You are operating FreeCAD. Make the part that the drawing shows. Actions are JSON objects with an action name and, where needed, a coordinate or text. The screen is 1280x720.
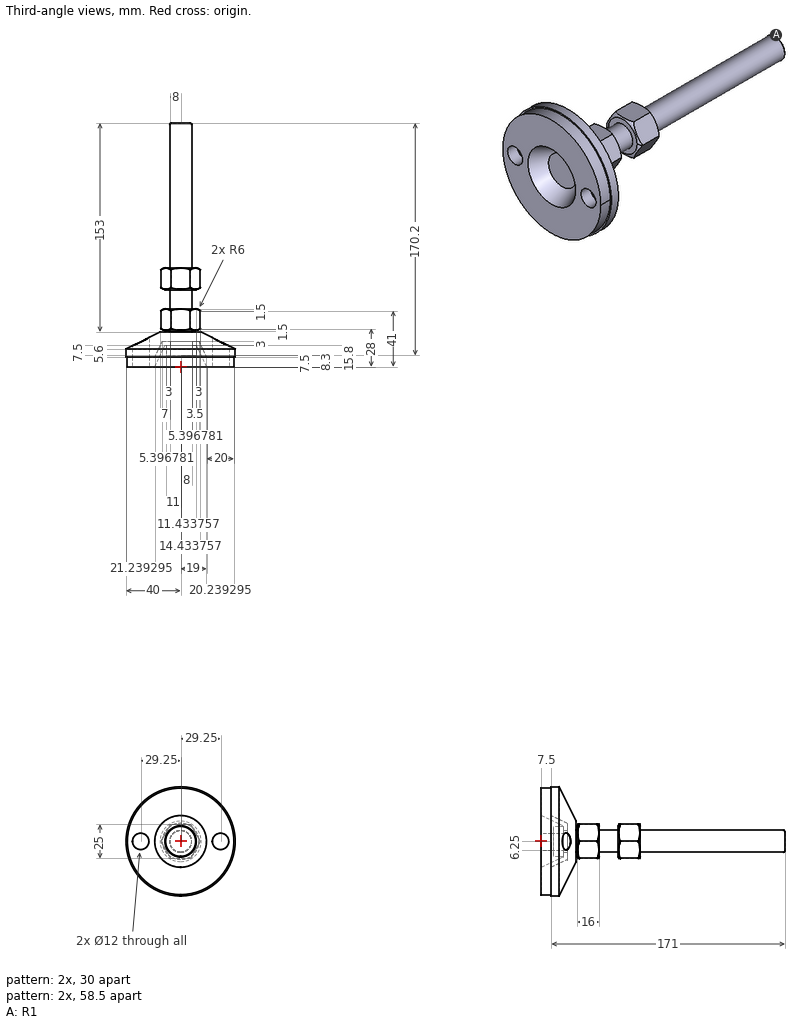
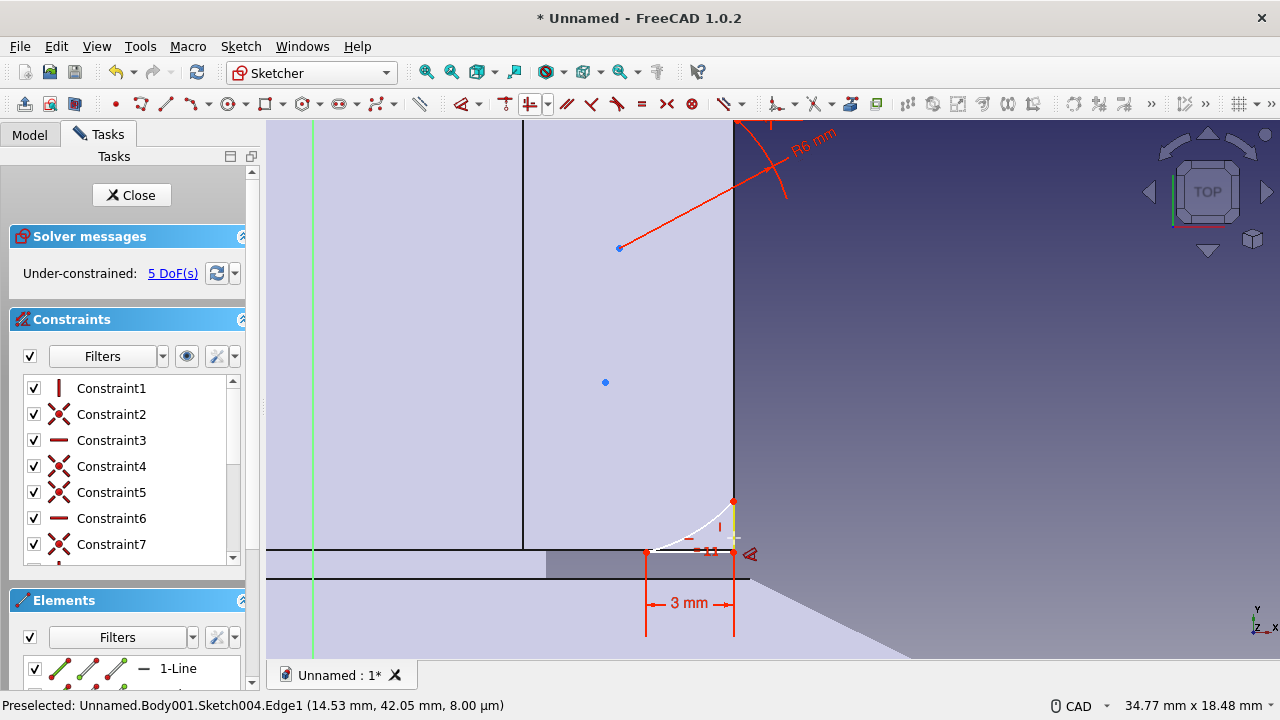
{"action": "left_click", "coordinate": [734, 537]}
{"action": "left_click", "coordinate": [768, 527]}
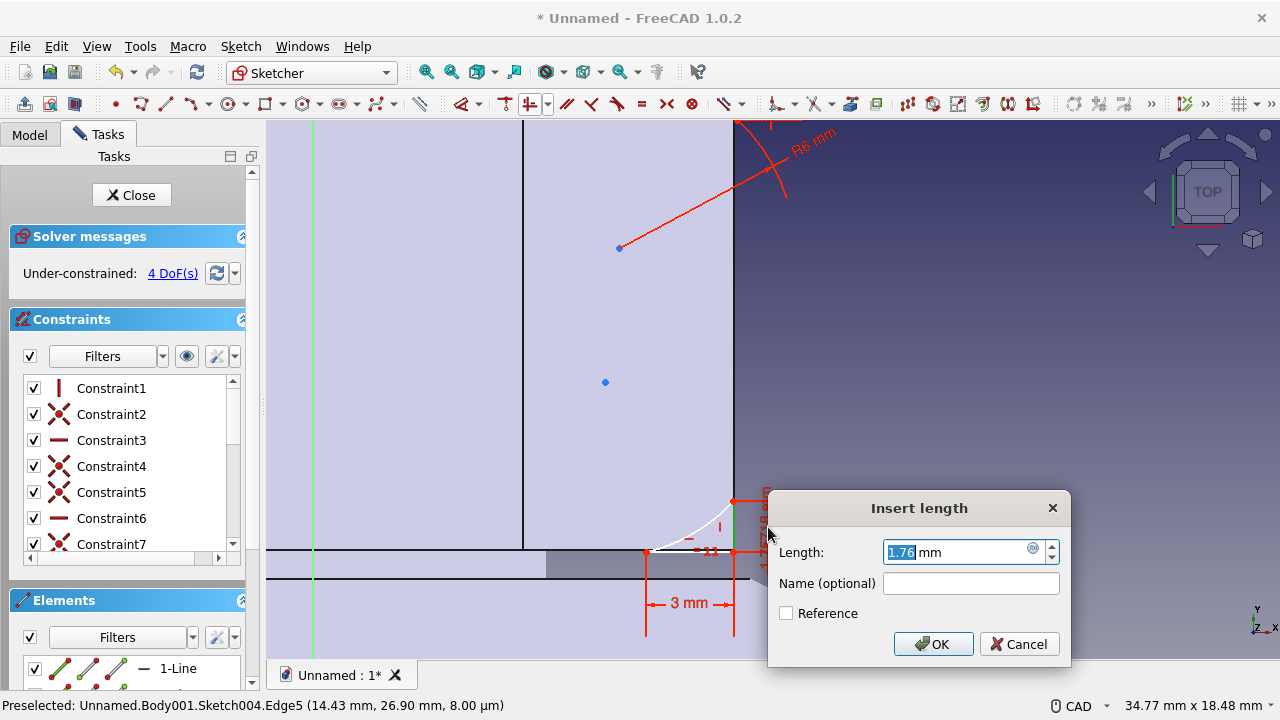
{"action": "type", "text": "1.5"}
{"action": "key", "text": "Return"}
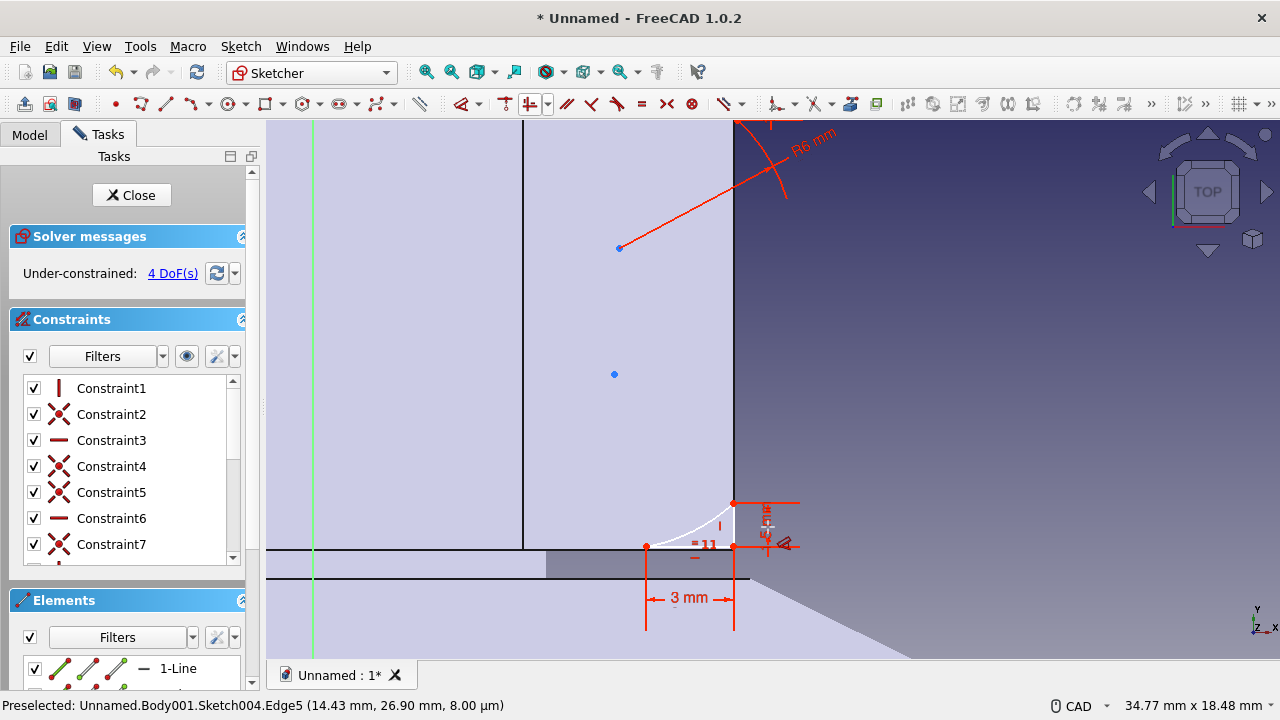
{"action": "scroll", "coordinate": [734, 538], "scroll_direction": "down", "scroll_amount": 2}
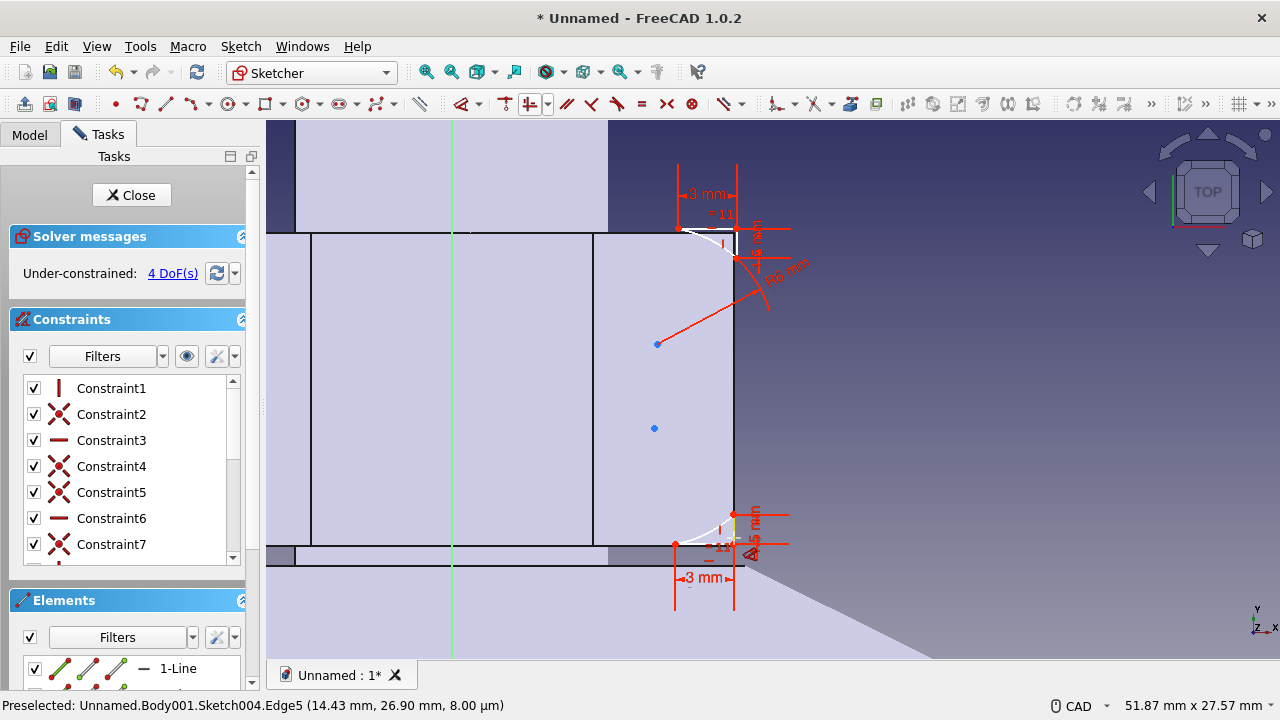
{"action": "left_click", "coordinate": [737, 258]}
{"action": "left_click", "coordinate": [418, 445]}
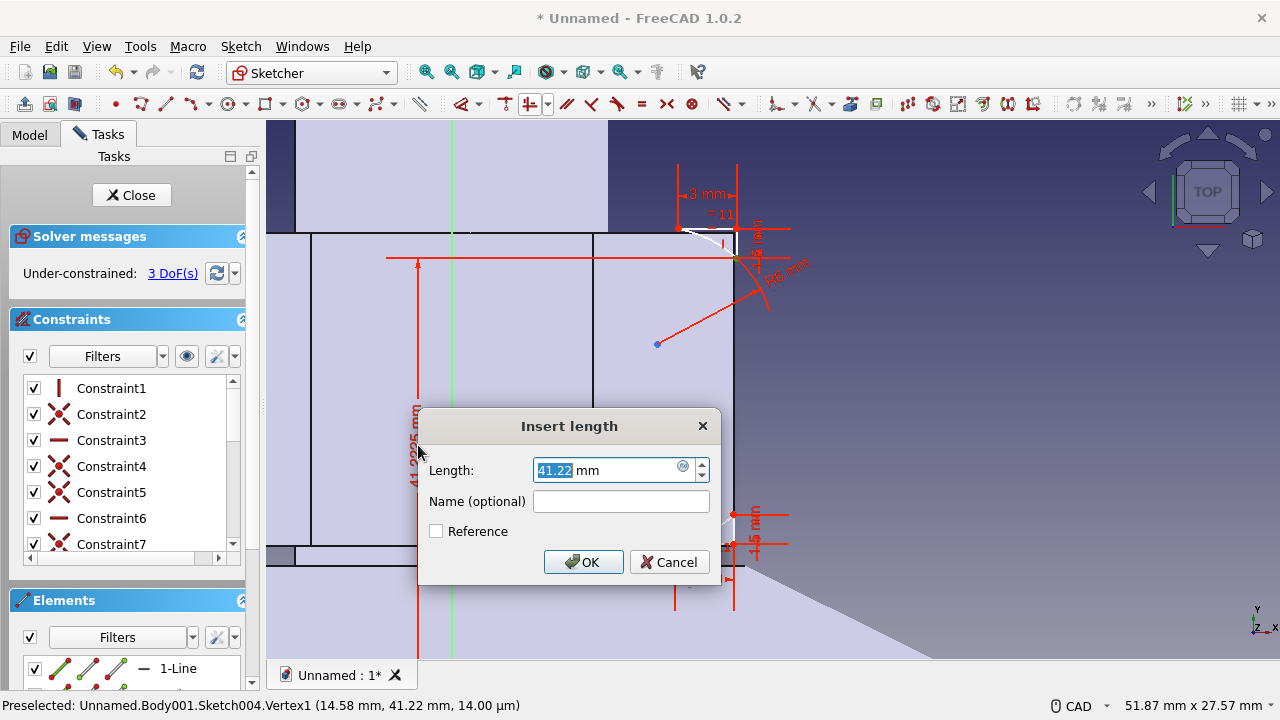
{"action": "type", "text": "41"}
{"action": "key", "text": "Return"}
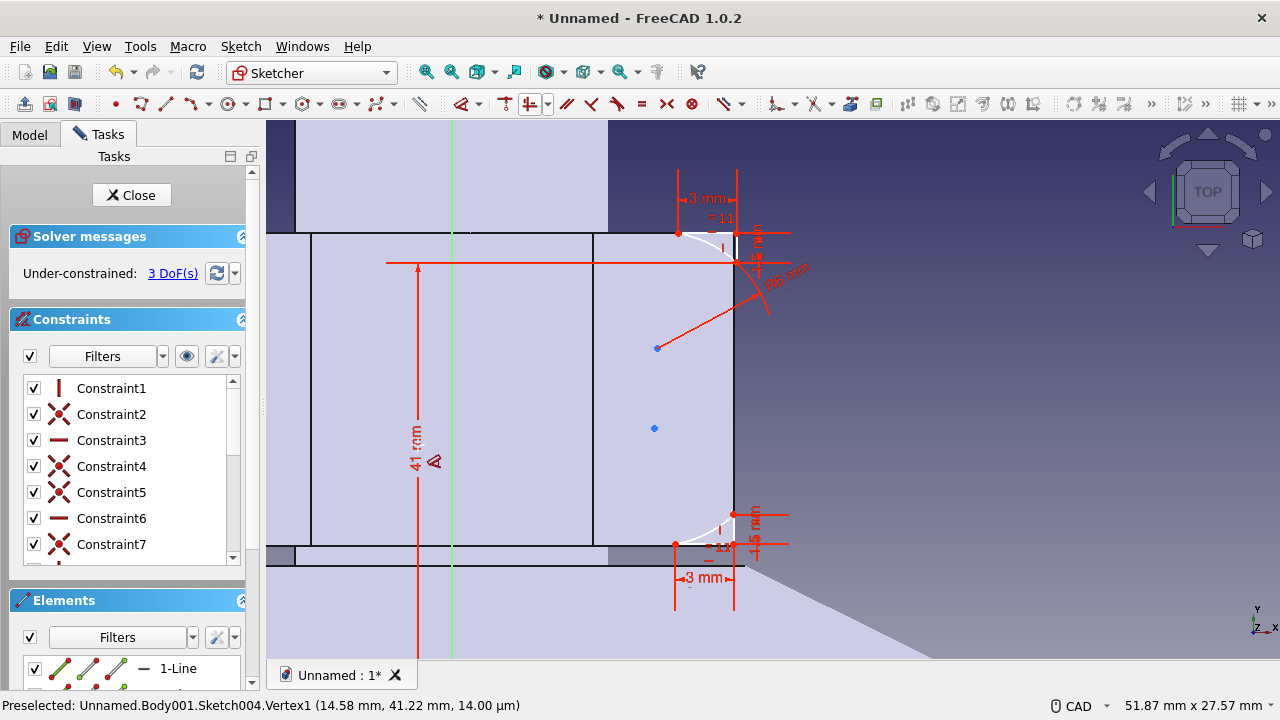
{"action": "left_click", "coordinate": [734, 515]}
{"action": "left_click", "coordinate": [418, 573]}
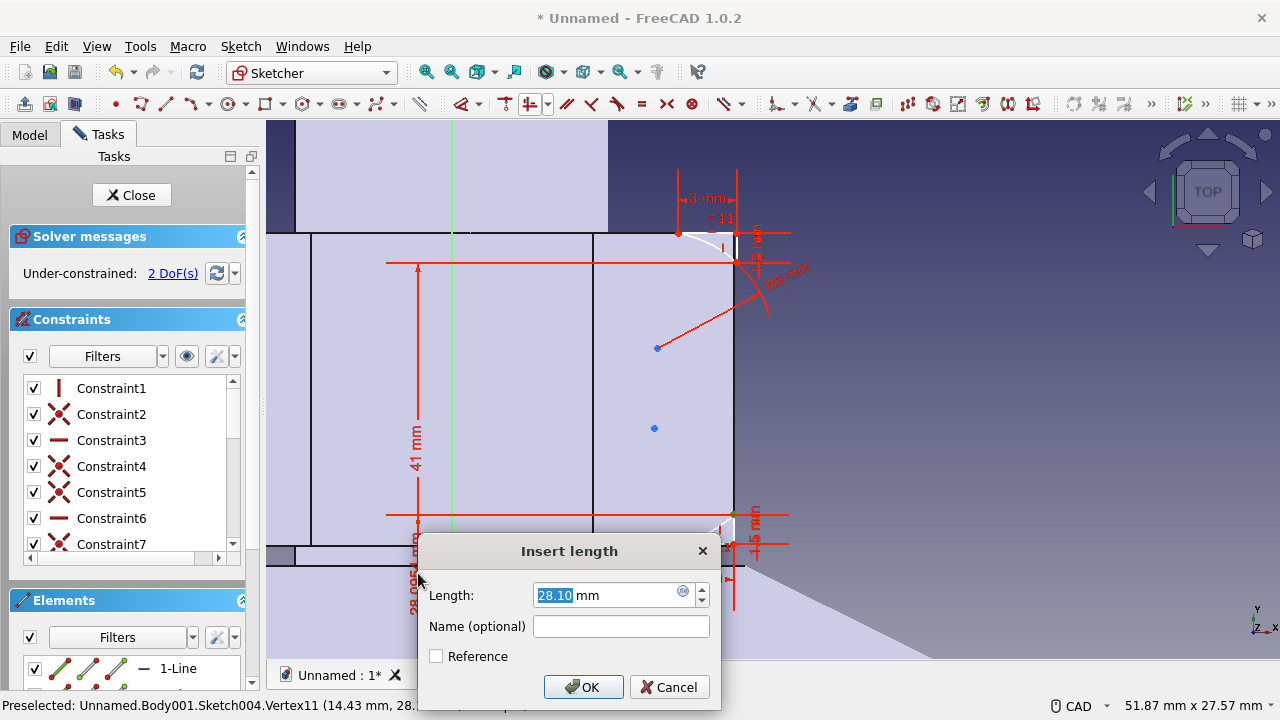
{"action": "type", "text": "28"}
{"action": "key", "text": "Return"}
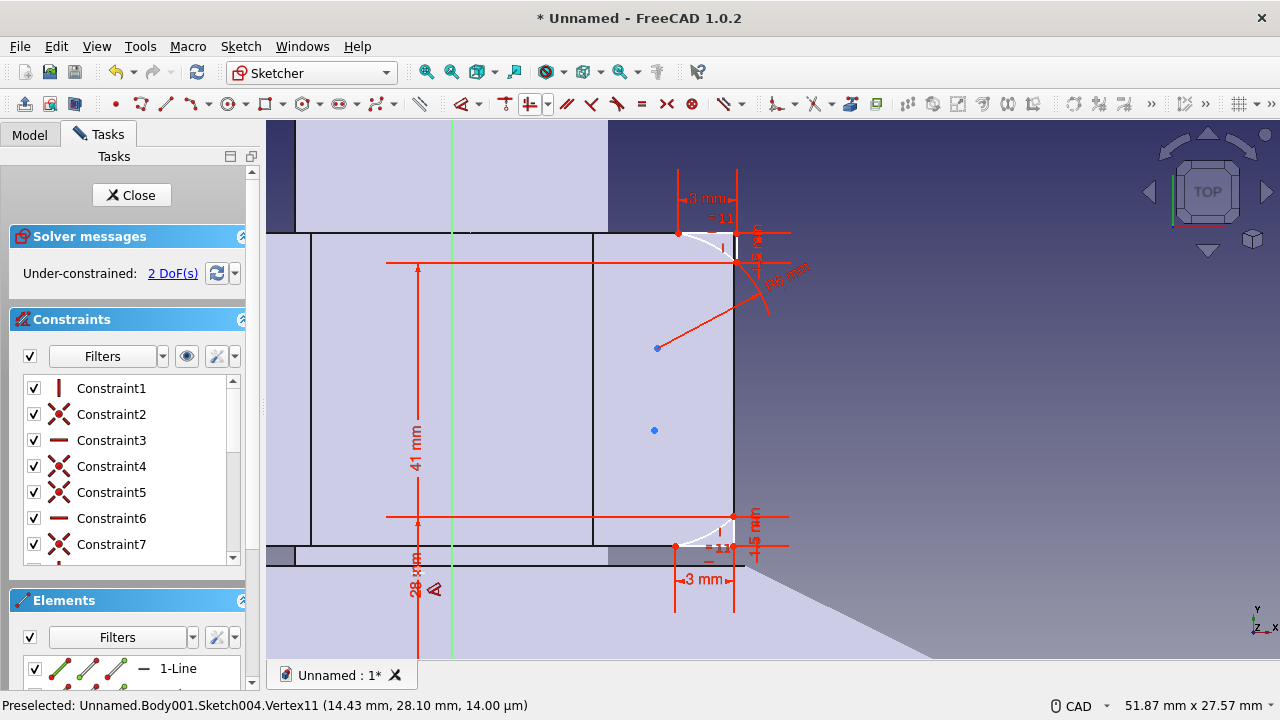
{"action": "left_click", "coordinate": [737, 263]}
{"action": "left_click", "coordinate": [594, 229]}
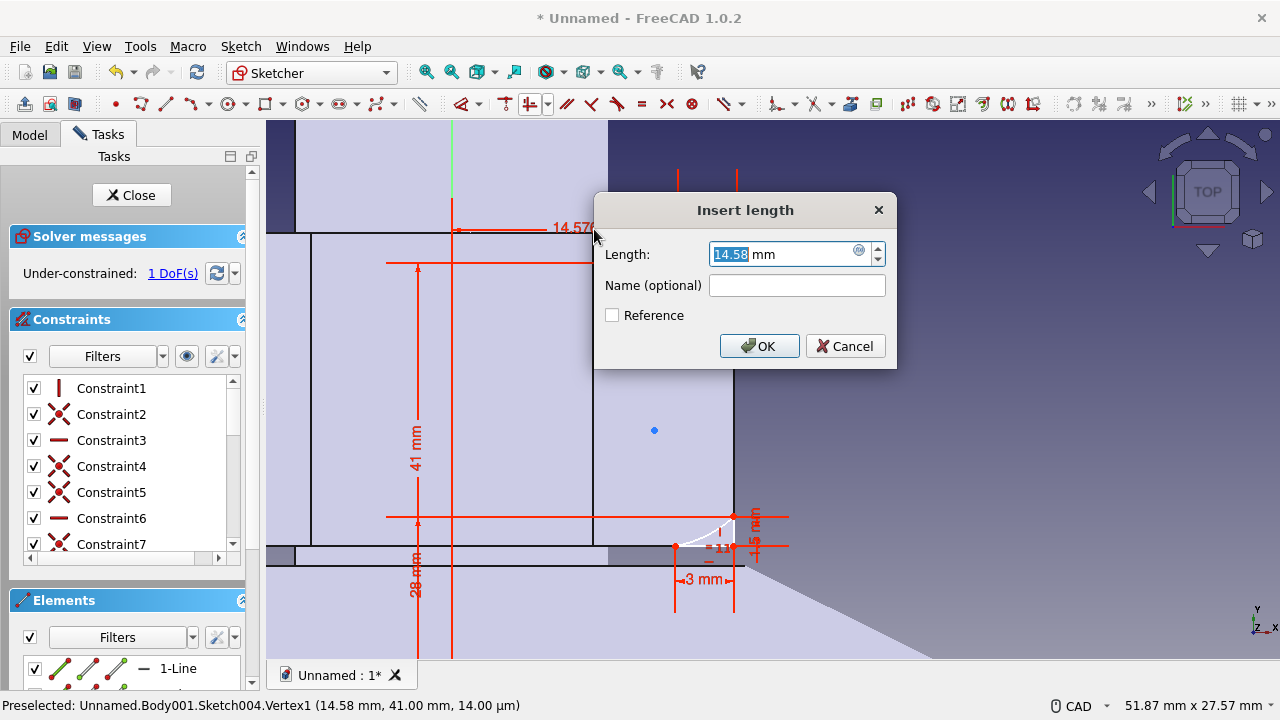
{"action": "type", "text": "14.433757"}
{"action": "key", "text": "Return"}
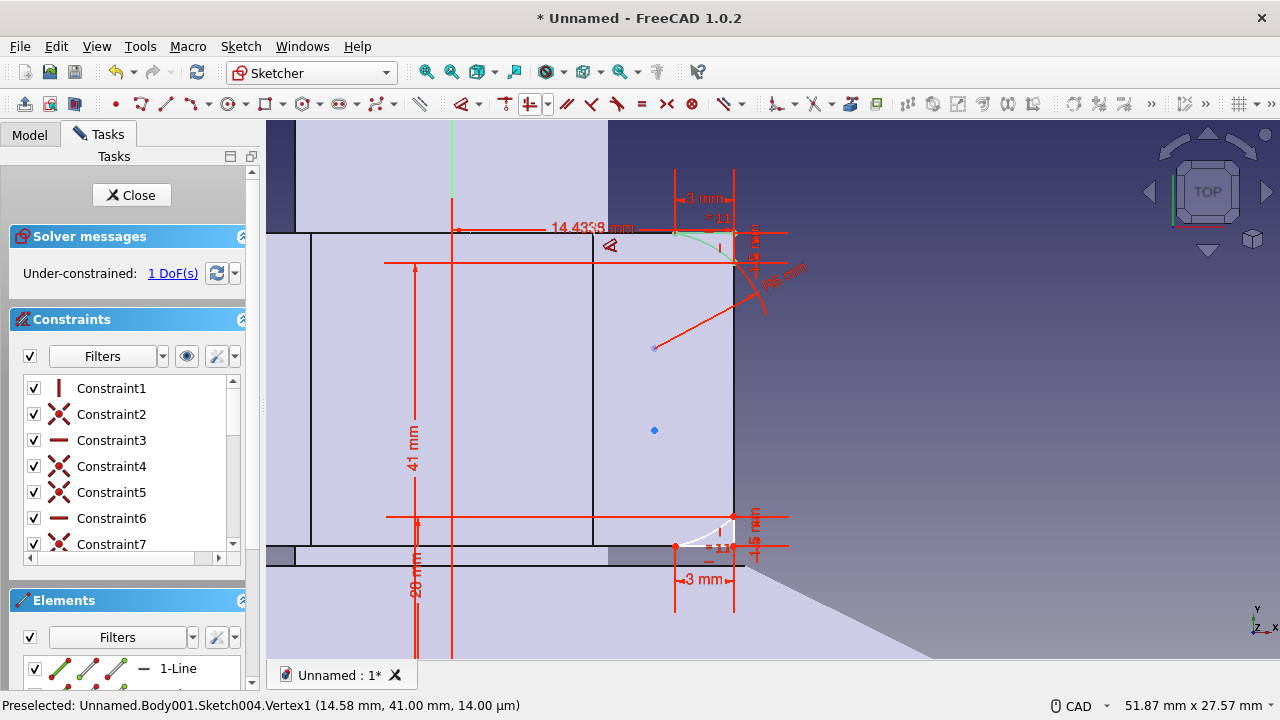
{"action": "left_click", "coordinate": [675, 546]}
{"action": "left_click", "coordinate": [564, 512]}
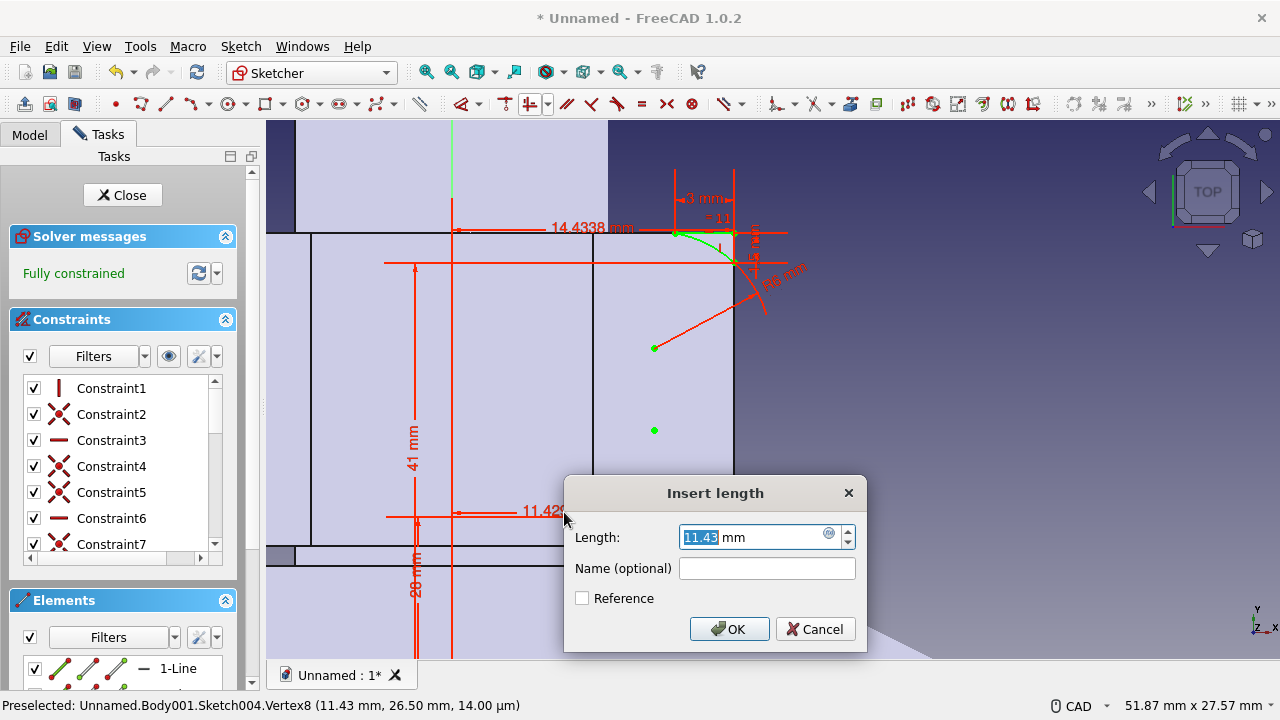
{"action": "type", "text": "11.433757"}
{"action": "key", "text": "Return"}
{"action": "key", "text": "Escape"}